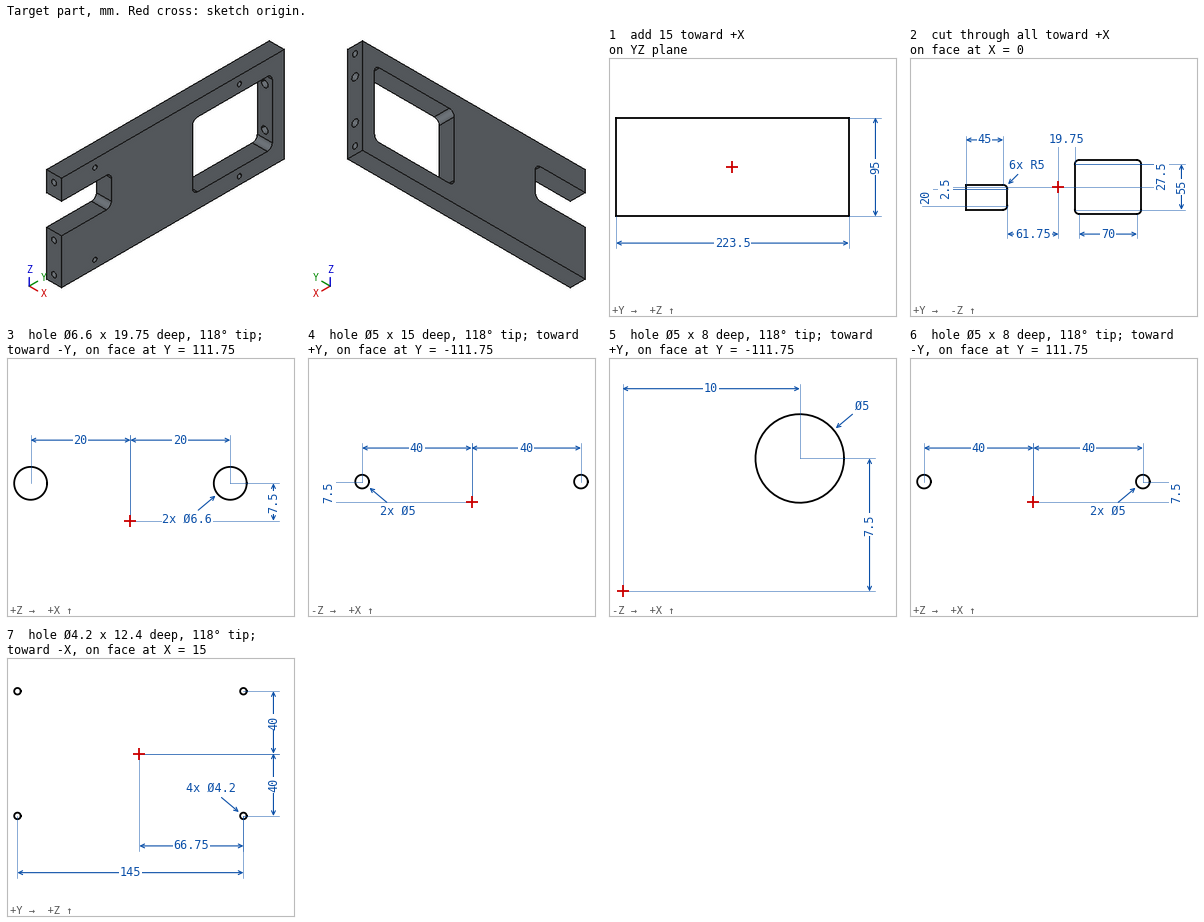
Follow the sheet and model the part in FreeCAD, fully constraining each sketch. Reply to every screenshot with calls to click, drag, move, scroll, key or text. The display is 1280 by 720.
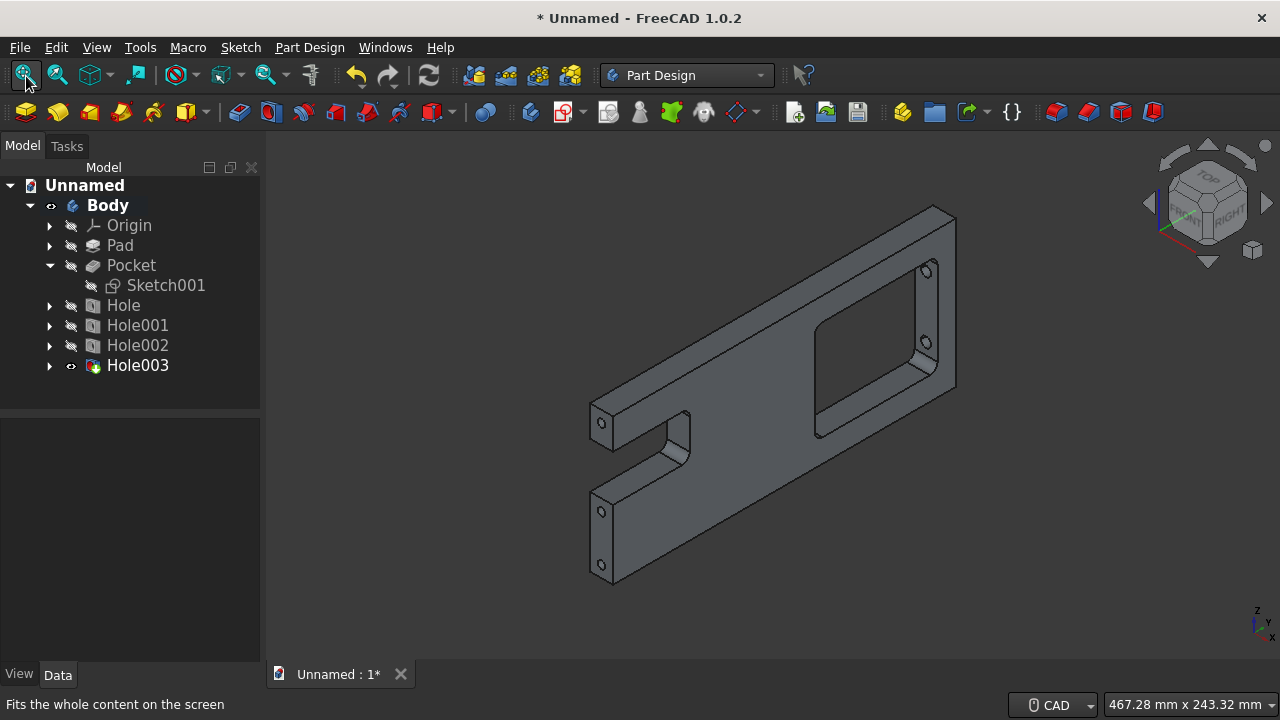
click(736, 453)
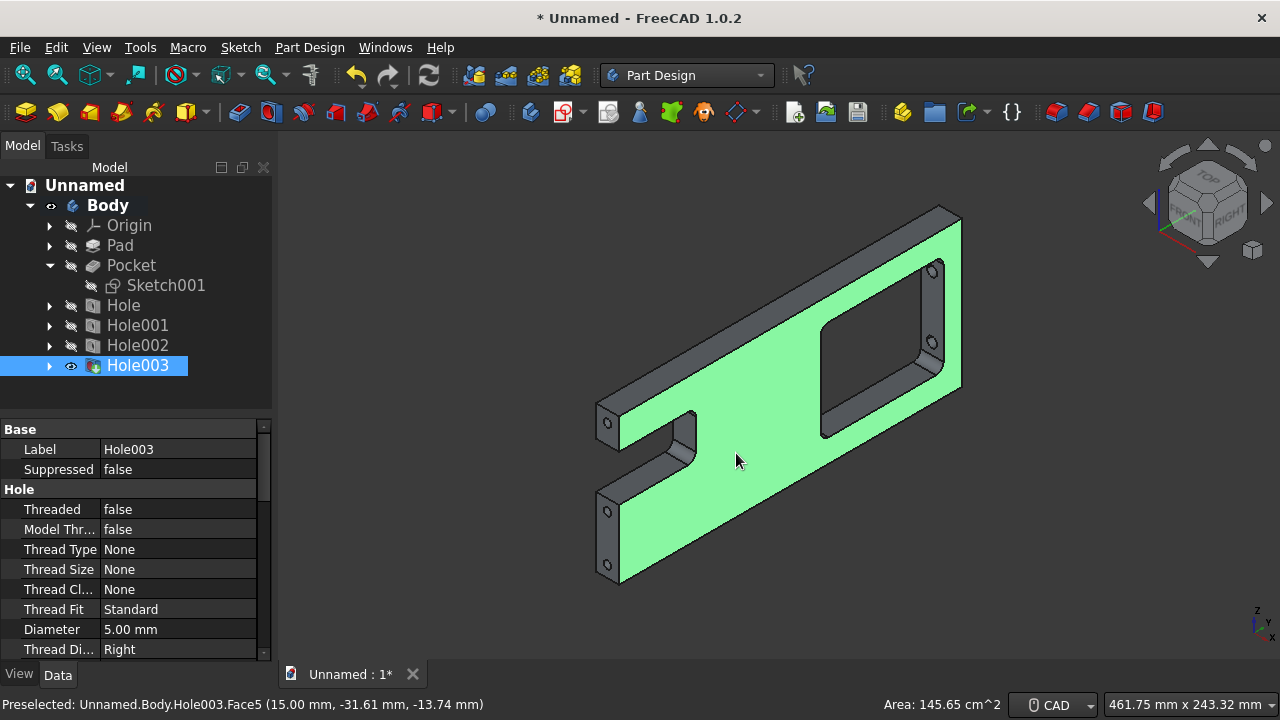
click(564, 112)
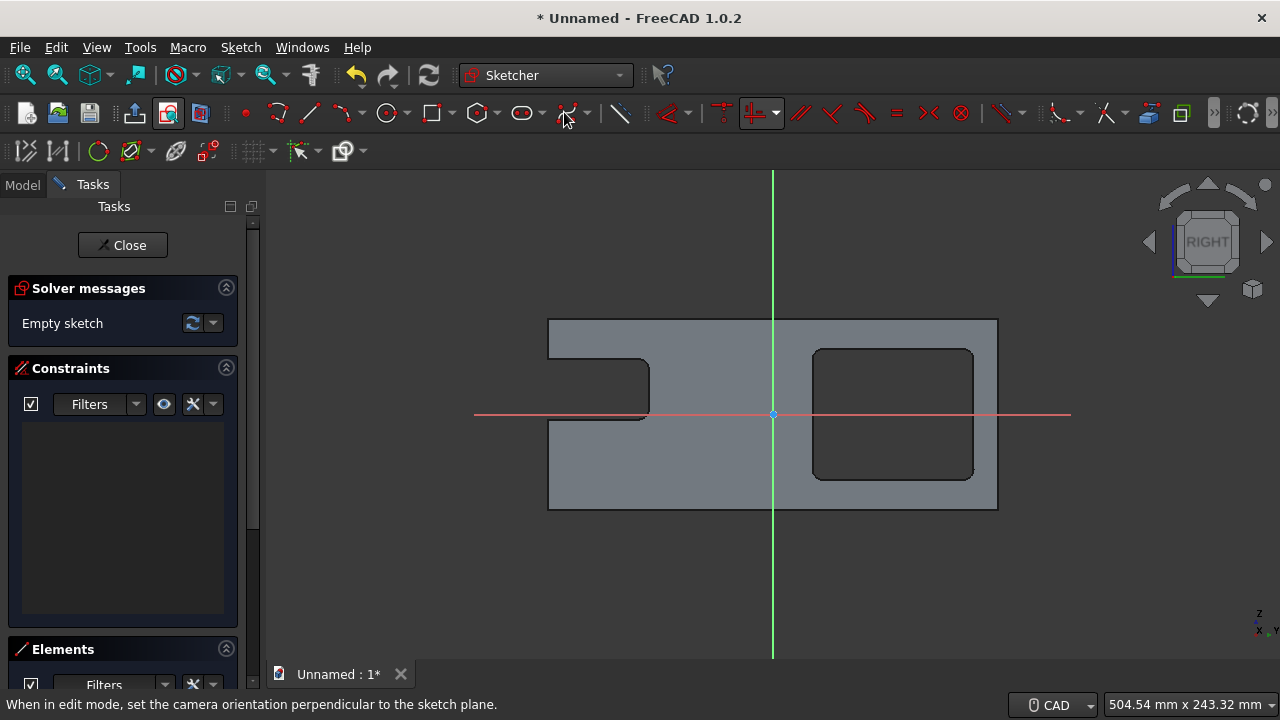
scroll(831, 415, up, 3)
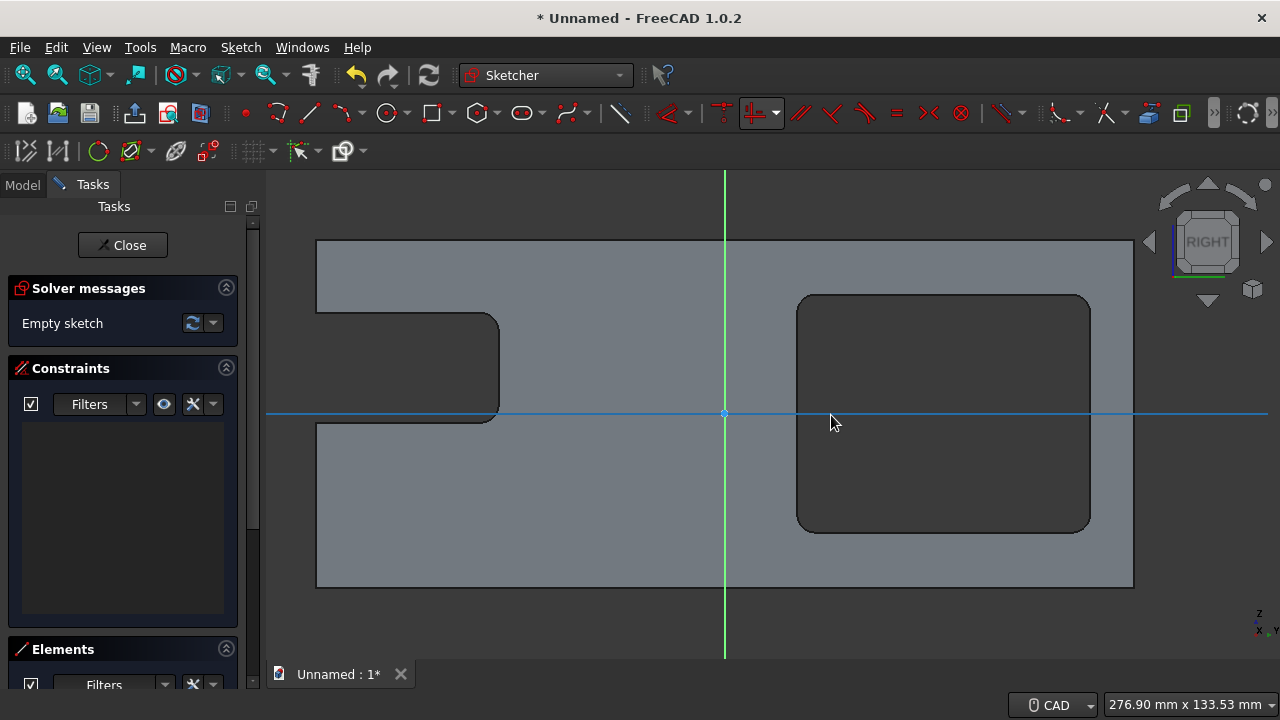
click(388, 114)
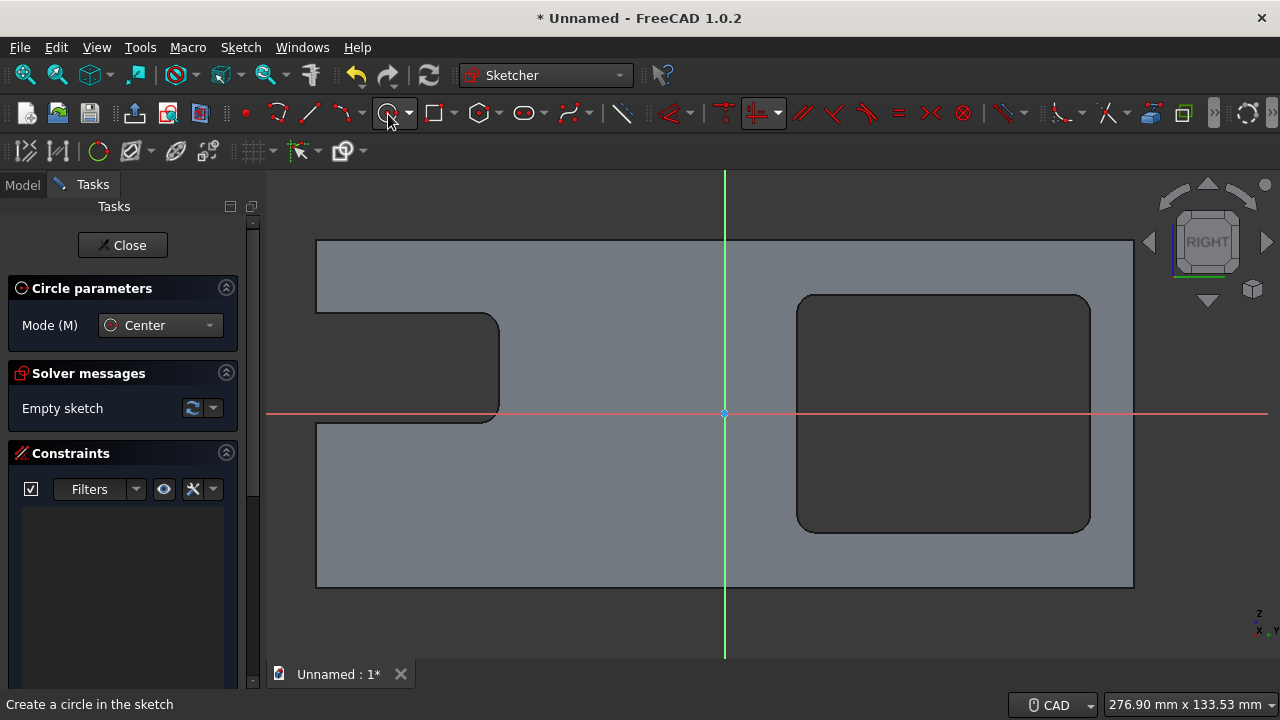
scroll(969, 560, up, 6)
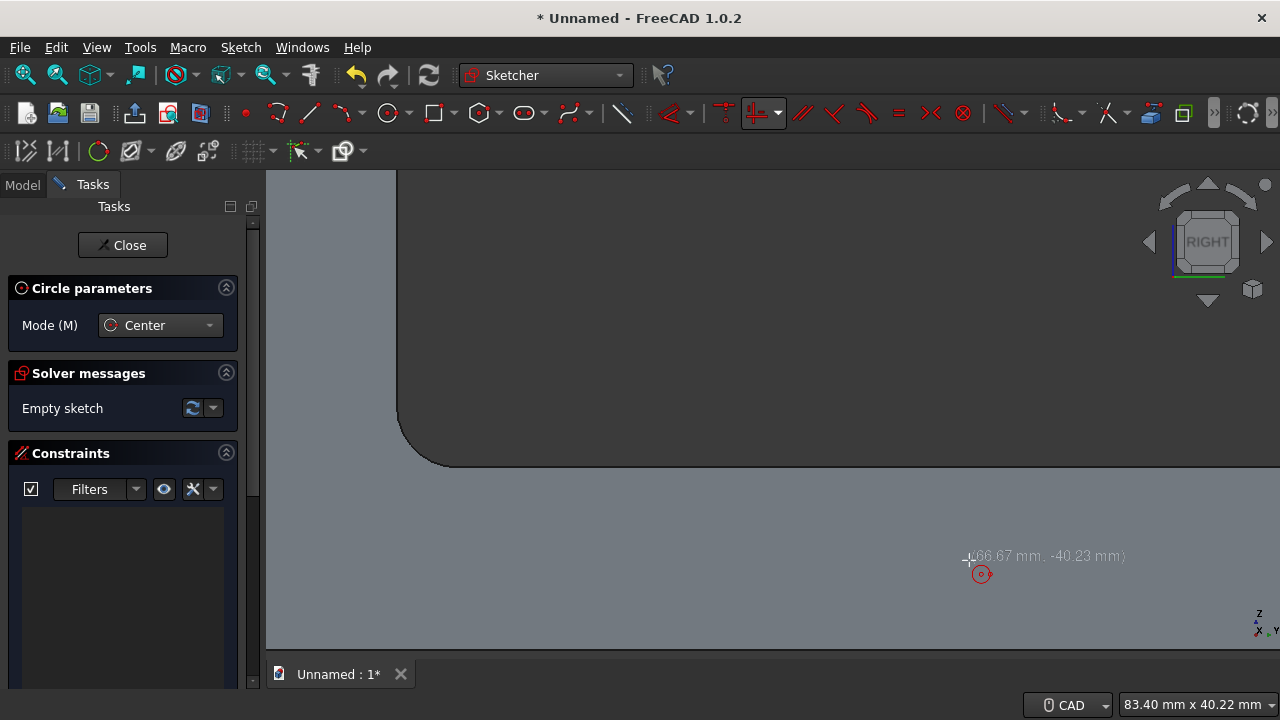
click(968, 559)
move(986, 541)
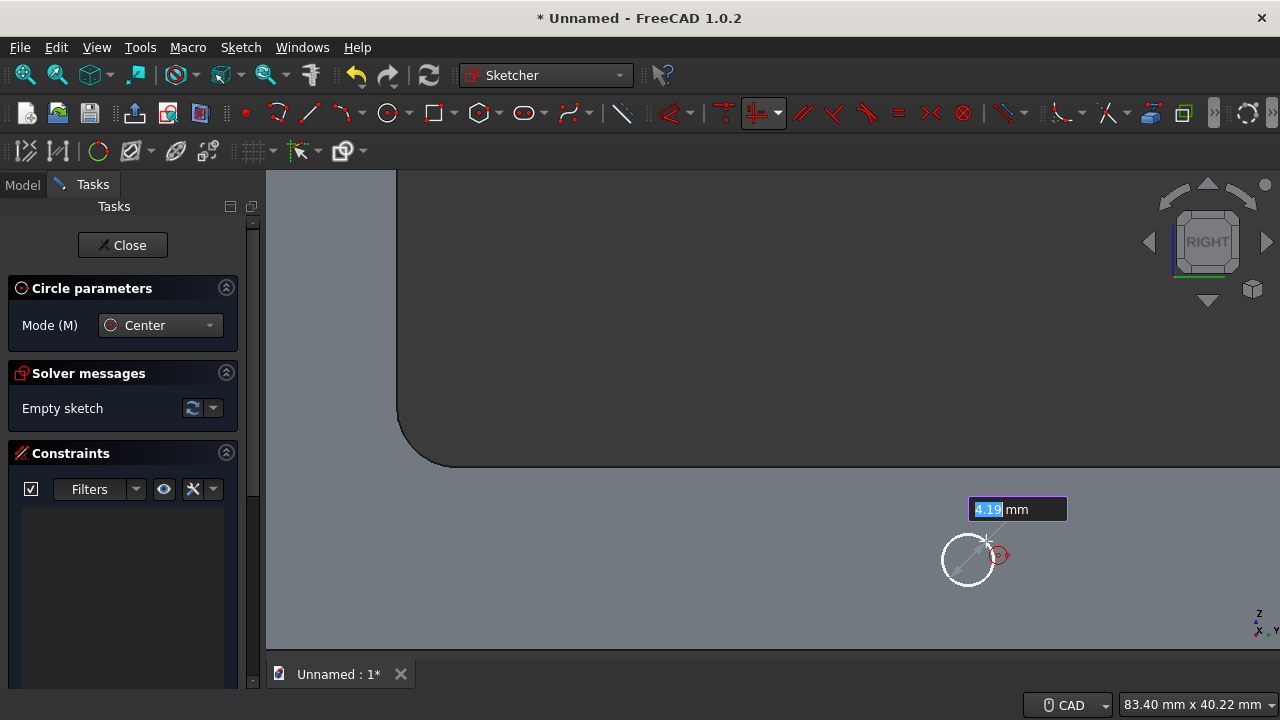
text(4.2)
key(Return)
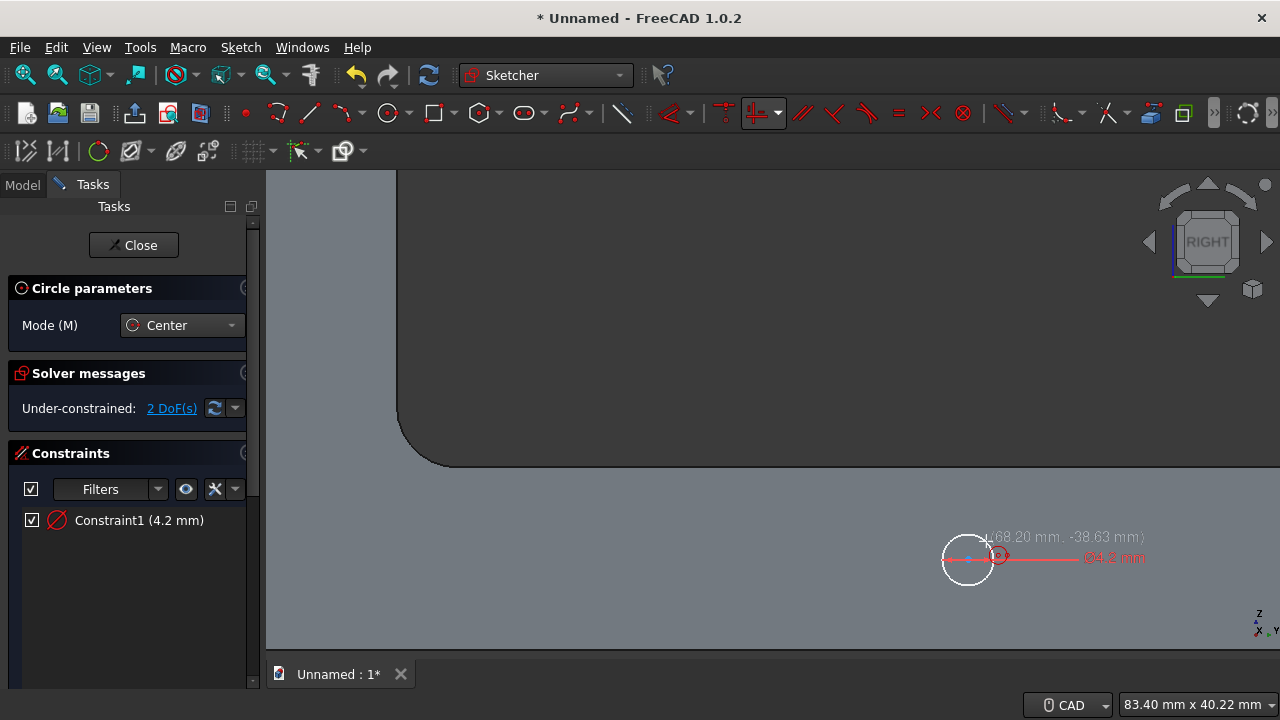
scroll(971, 562, down, 6)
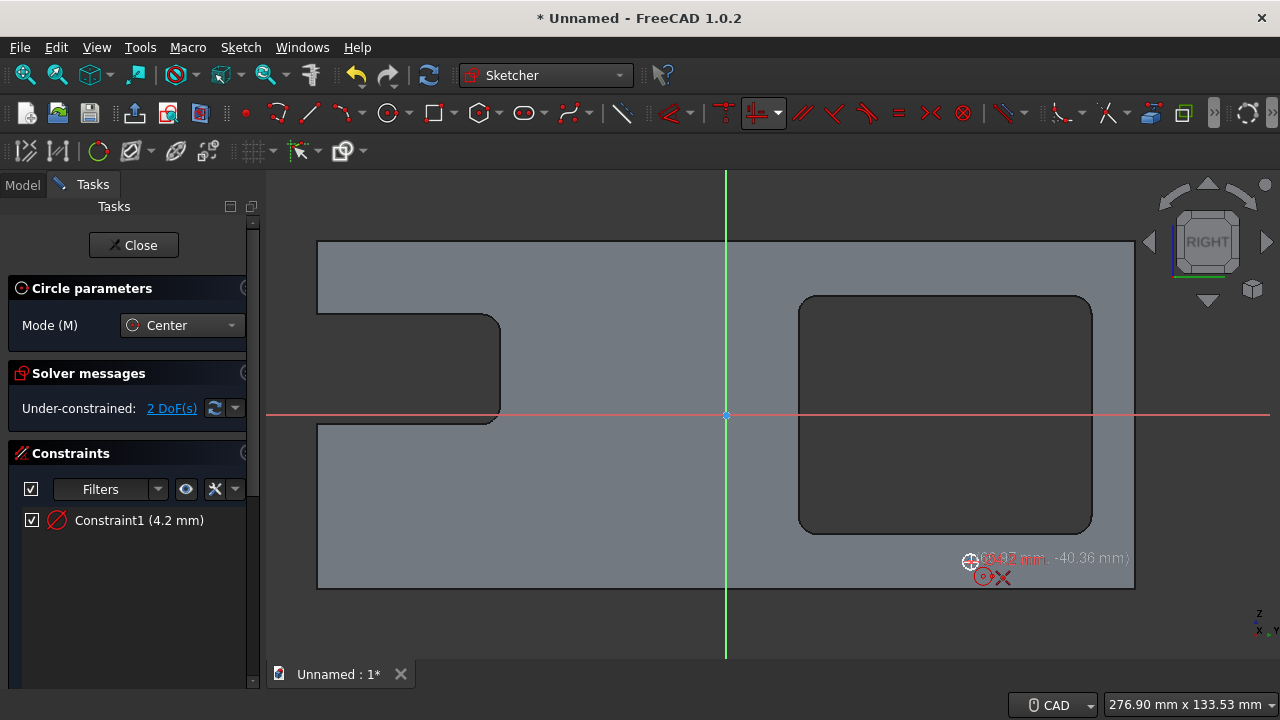
scroll(971, 269, up, 6)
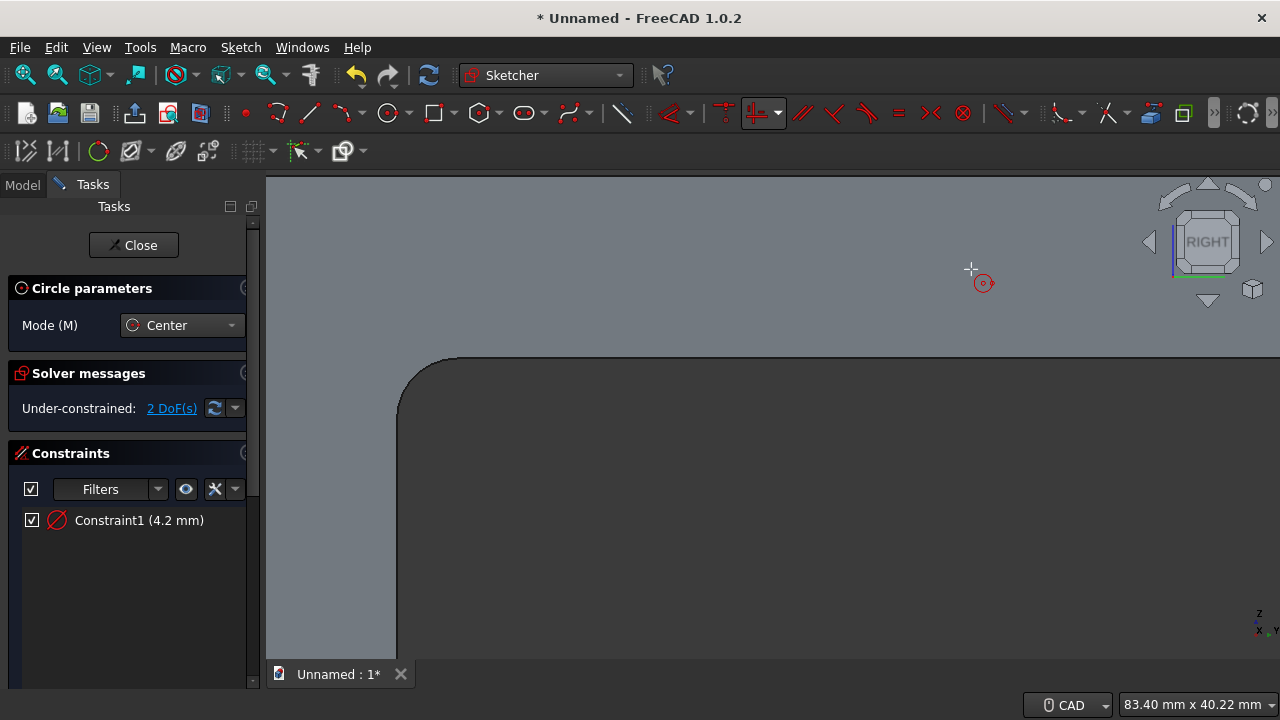
click(968, 267)
move(986, 249)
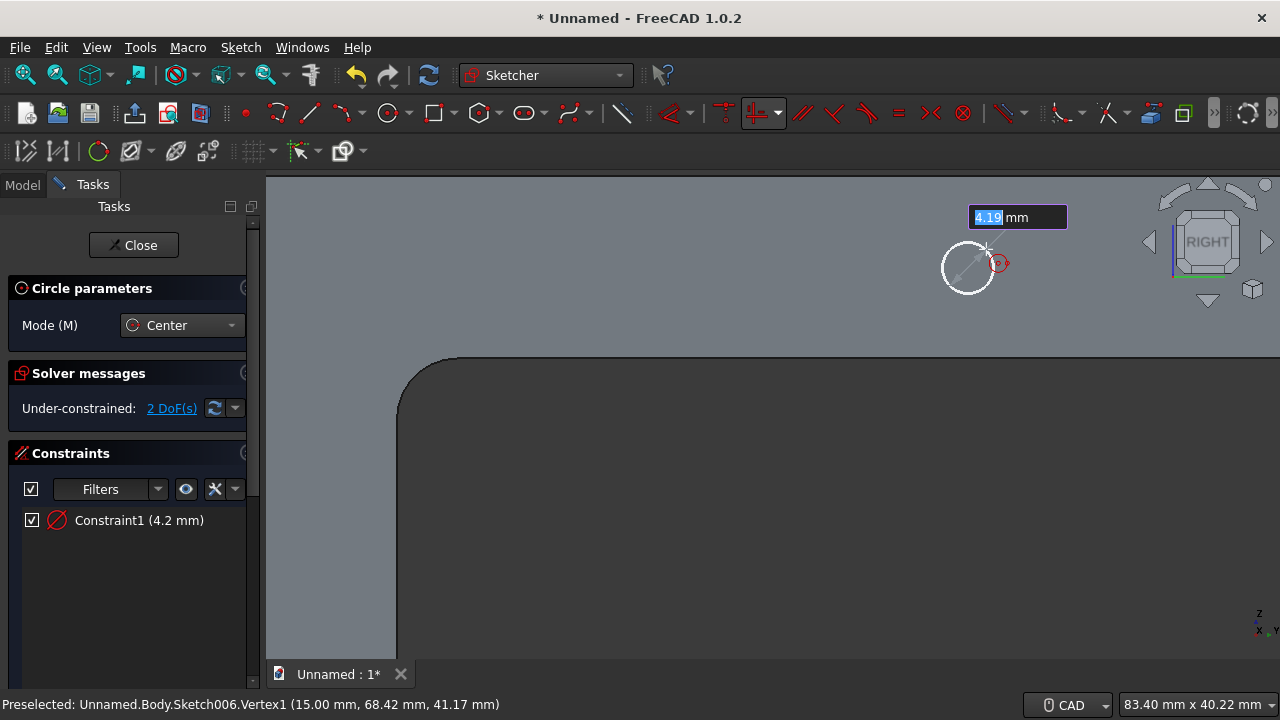
text(4.2)
key(Return)